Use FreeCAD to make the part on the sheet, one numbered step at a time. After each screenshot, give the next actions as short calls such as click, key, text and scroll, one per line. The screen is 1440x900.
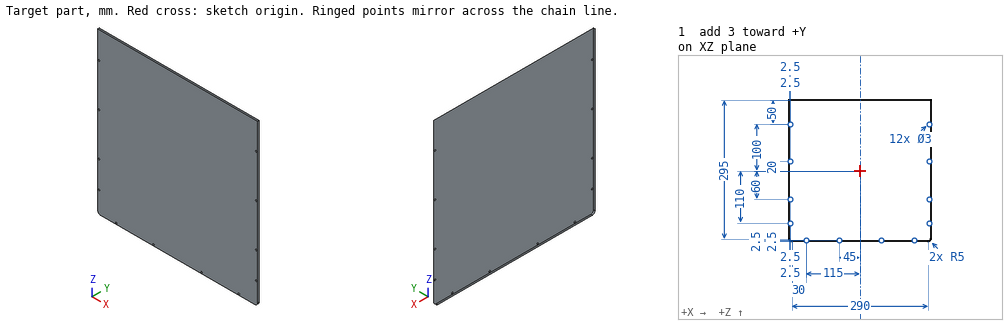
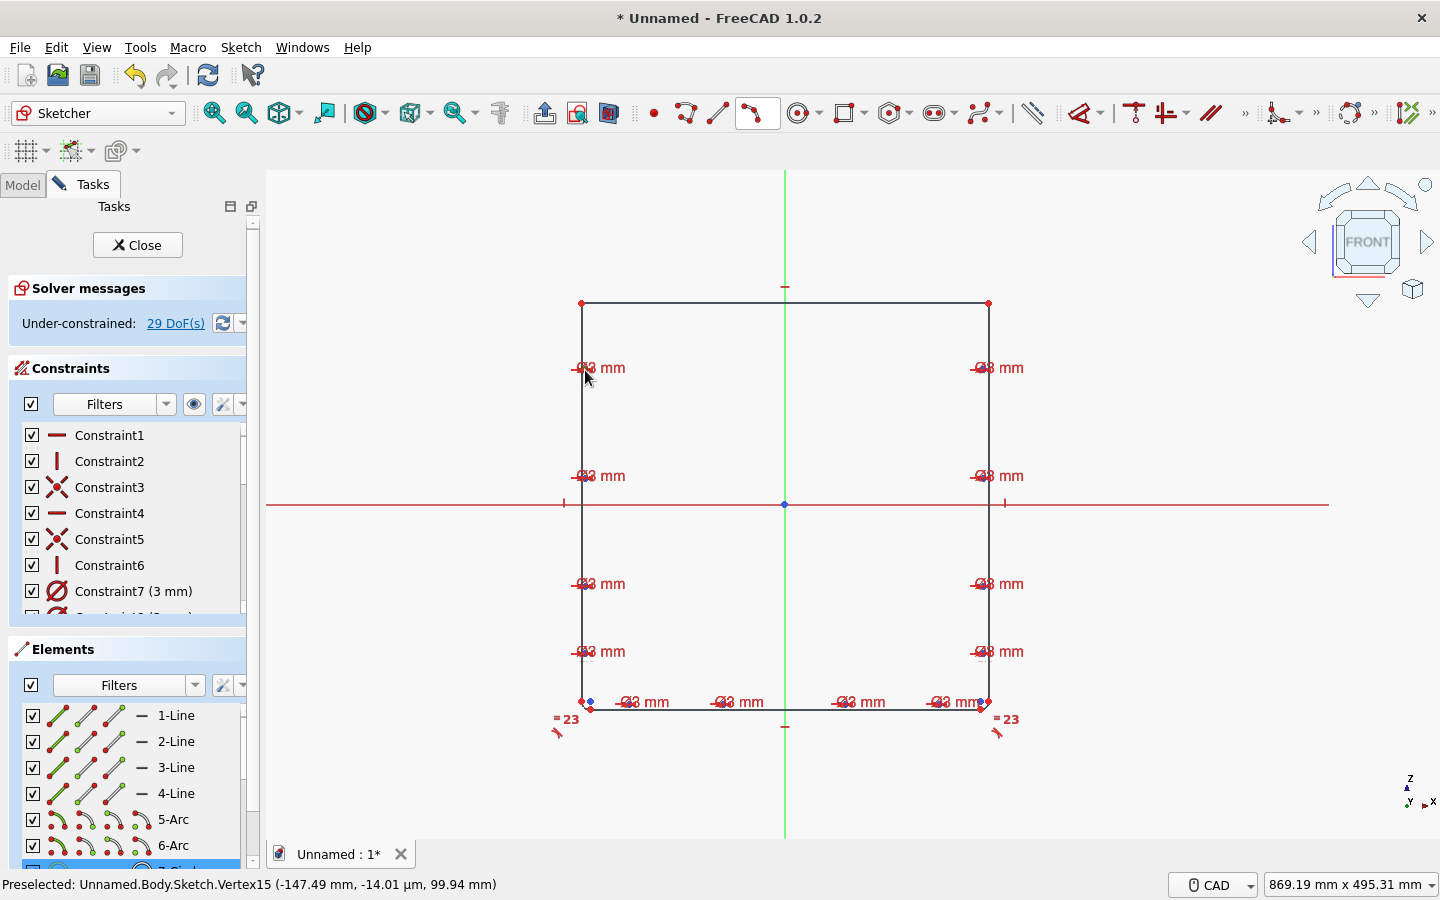
click(984, 370)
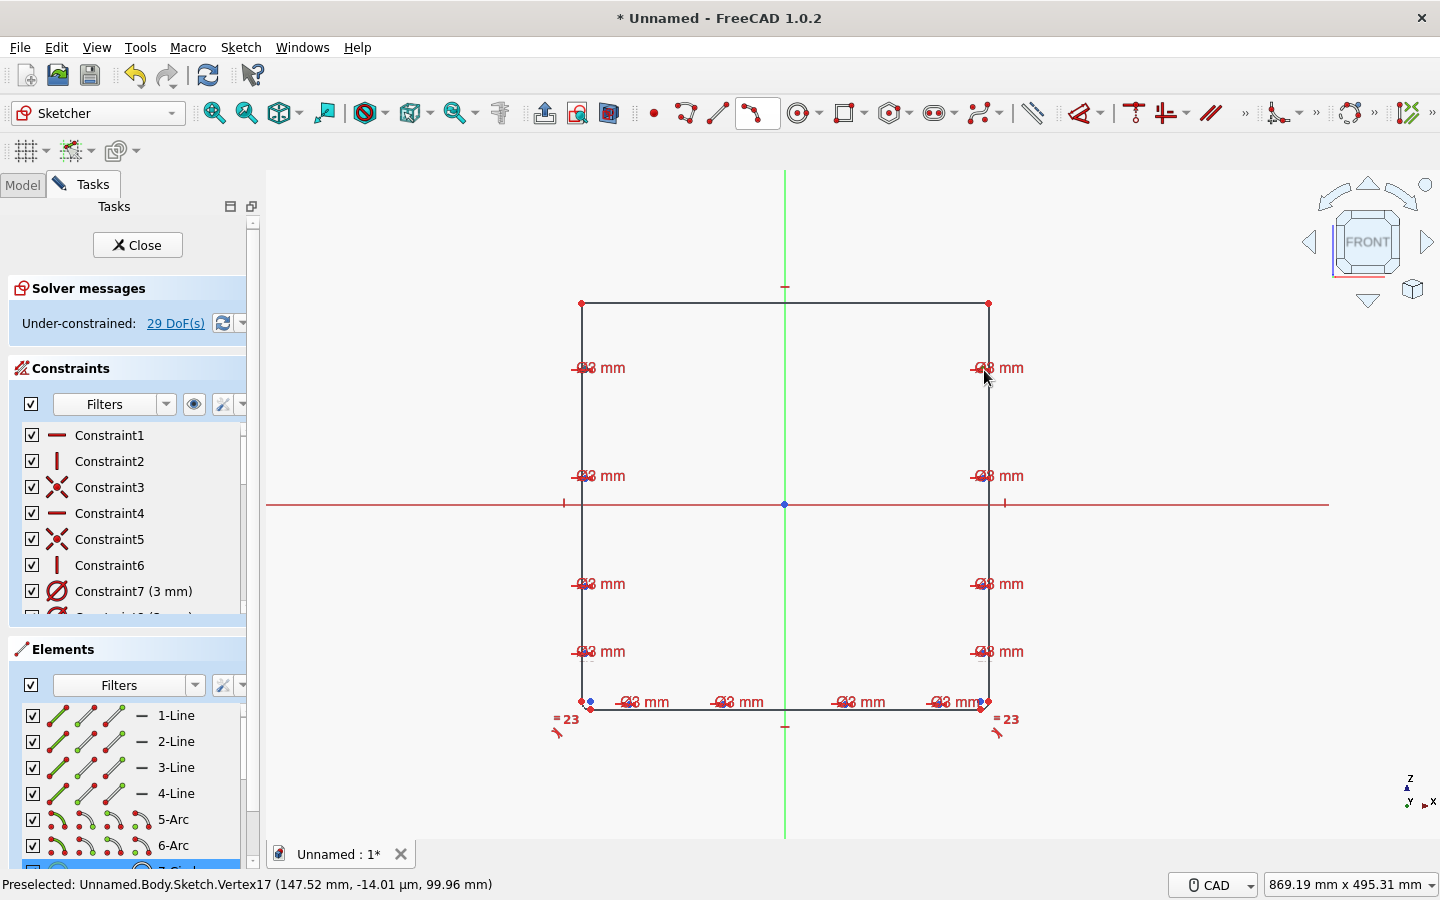
click(785, 767)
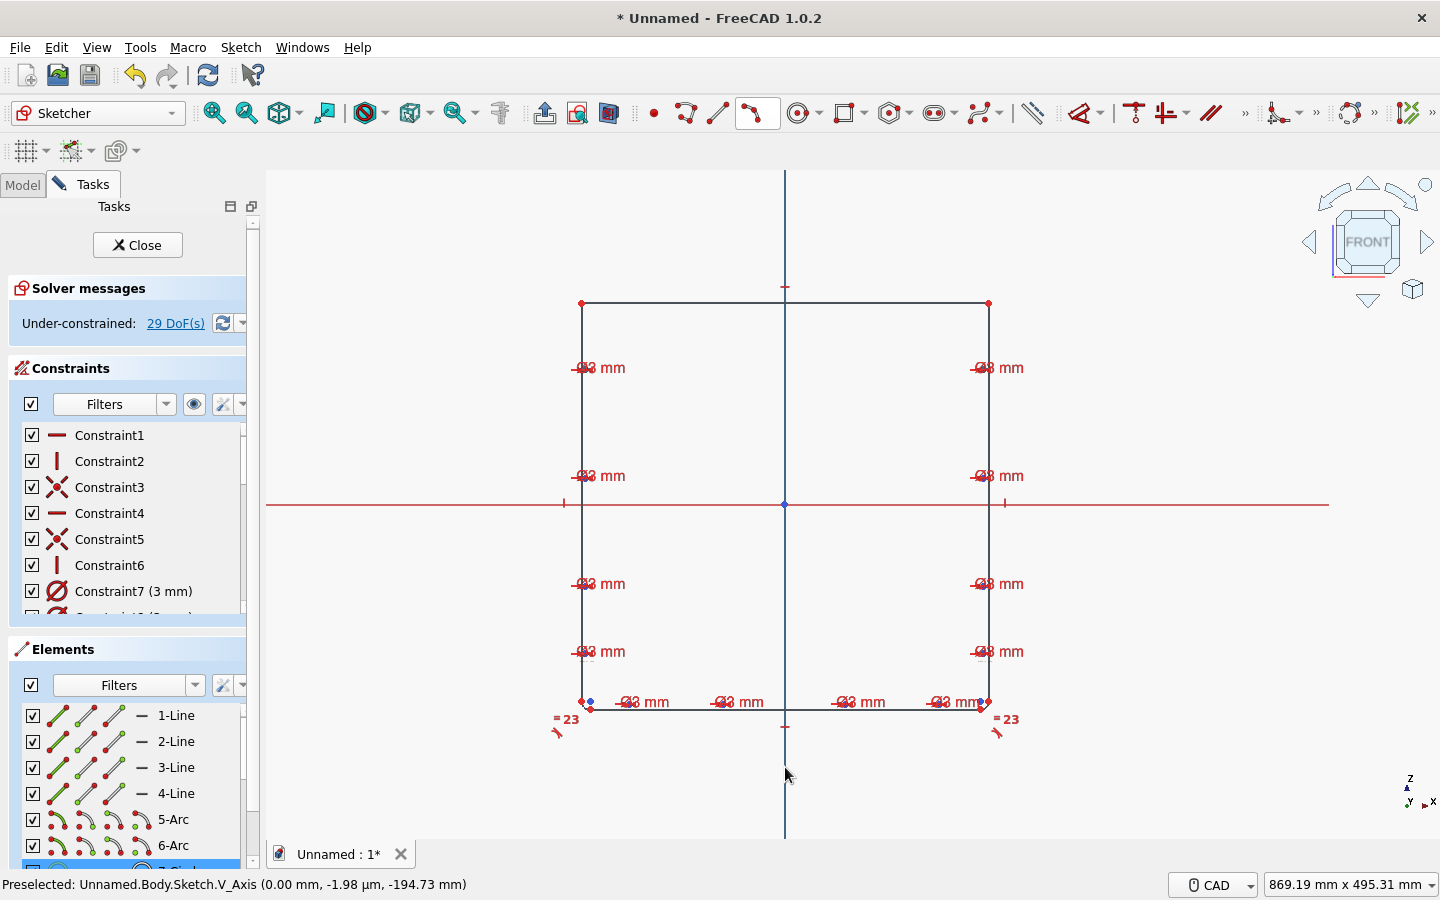
key(s)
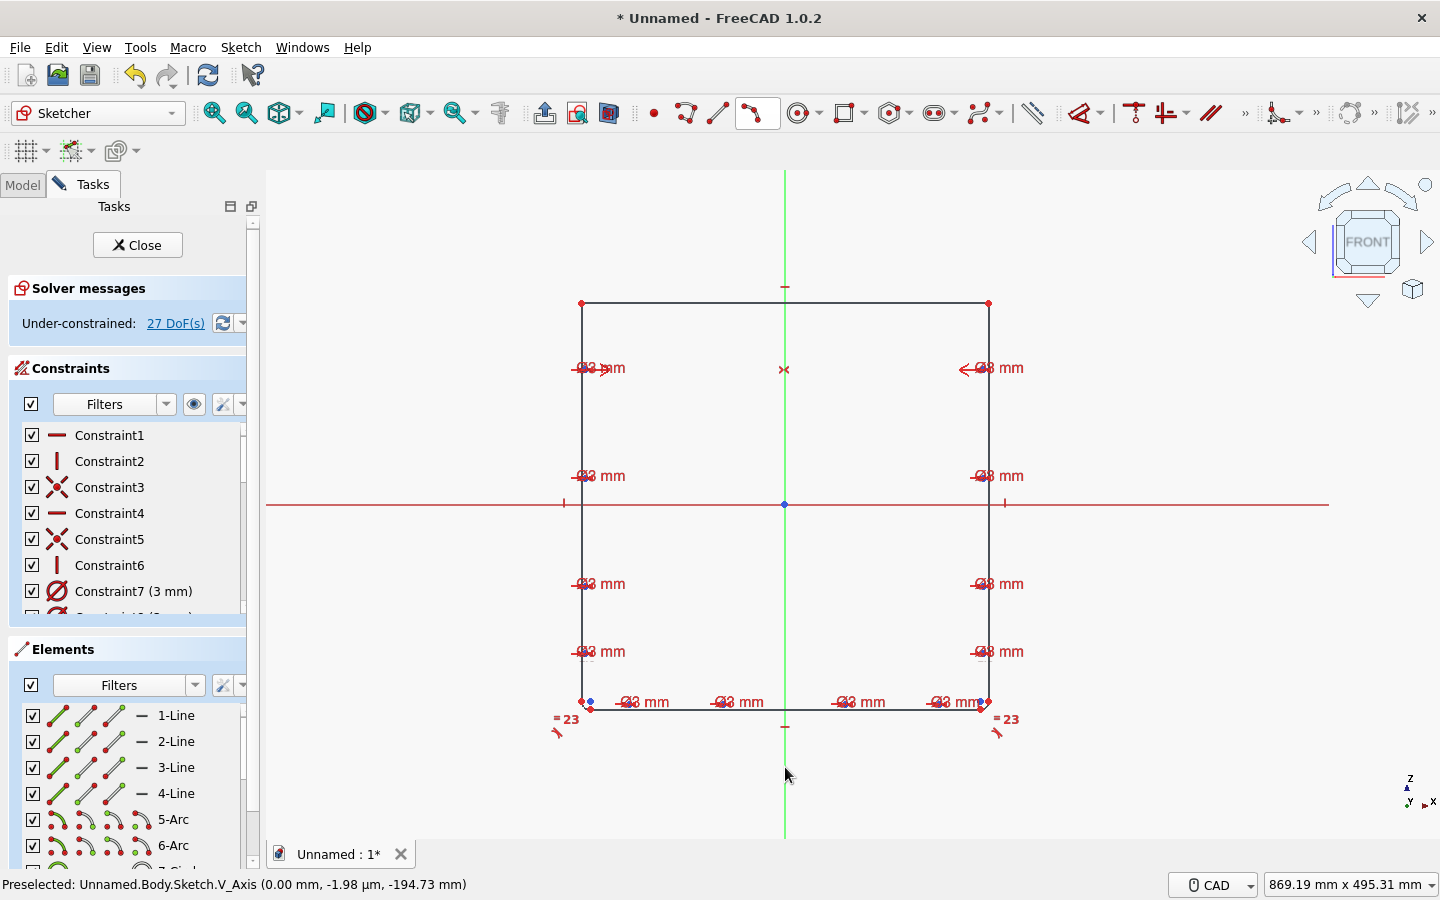
click(585, 478)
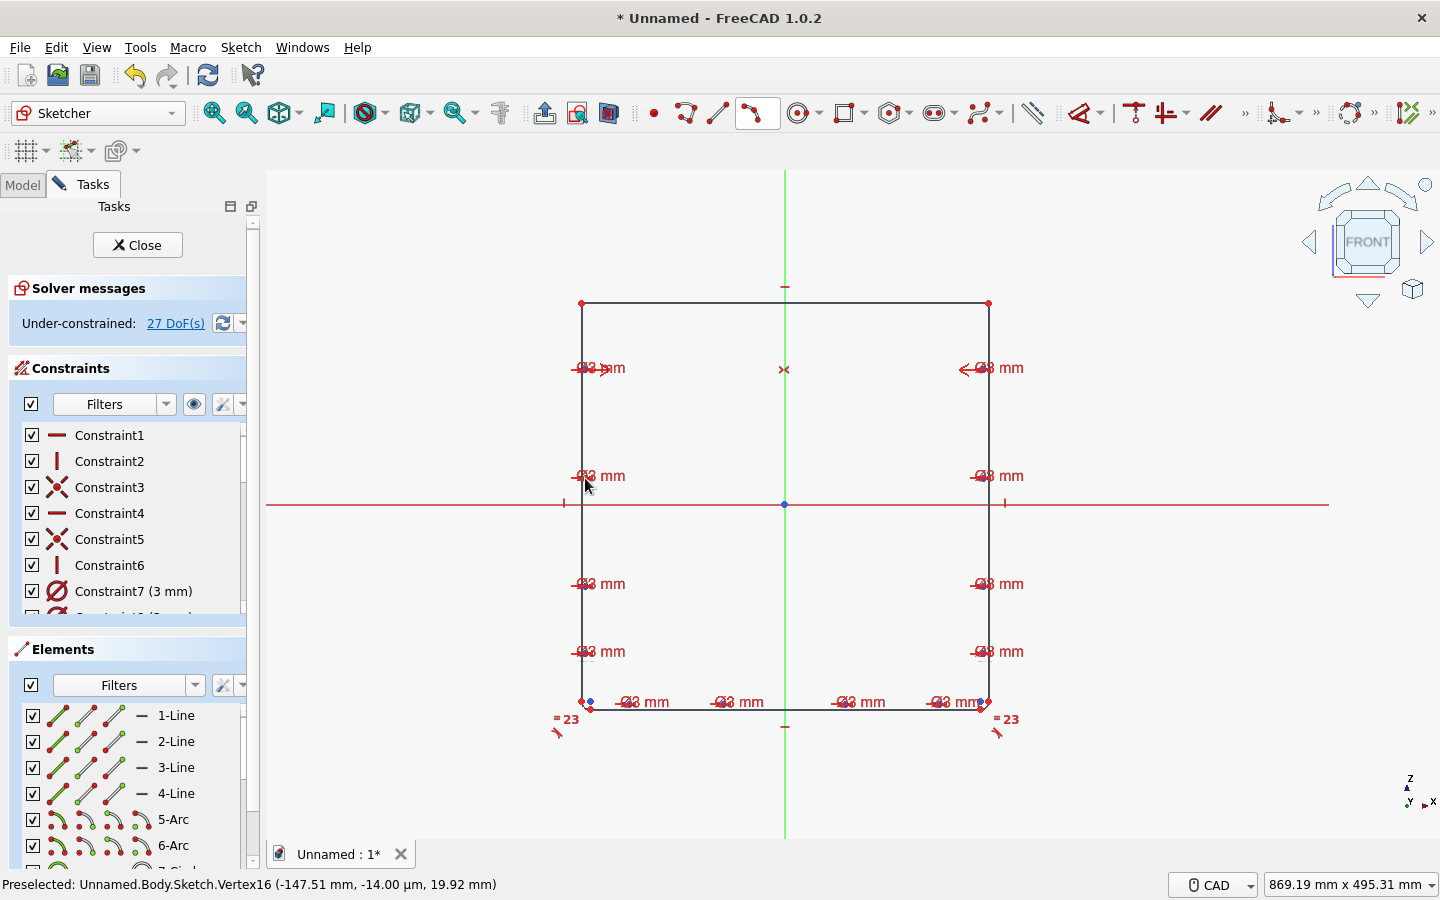
click(984, 478)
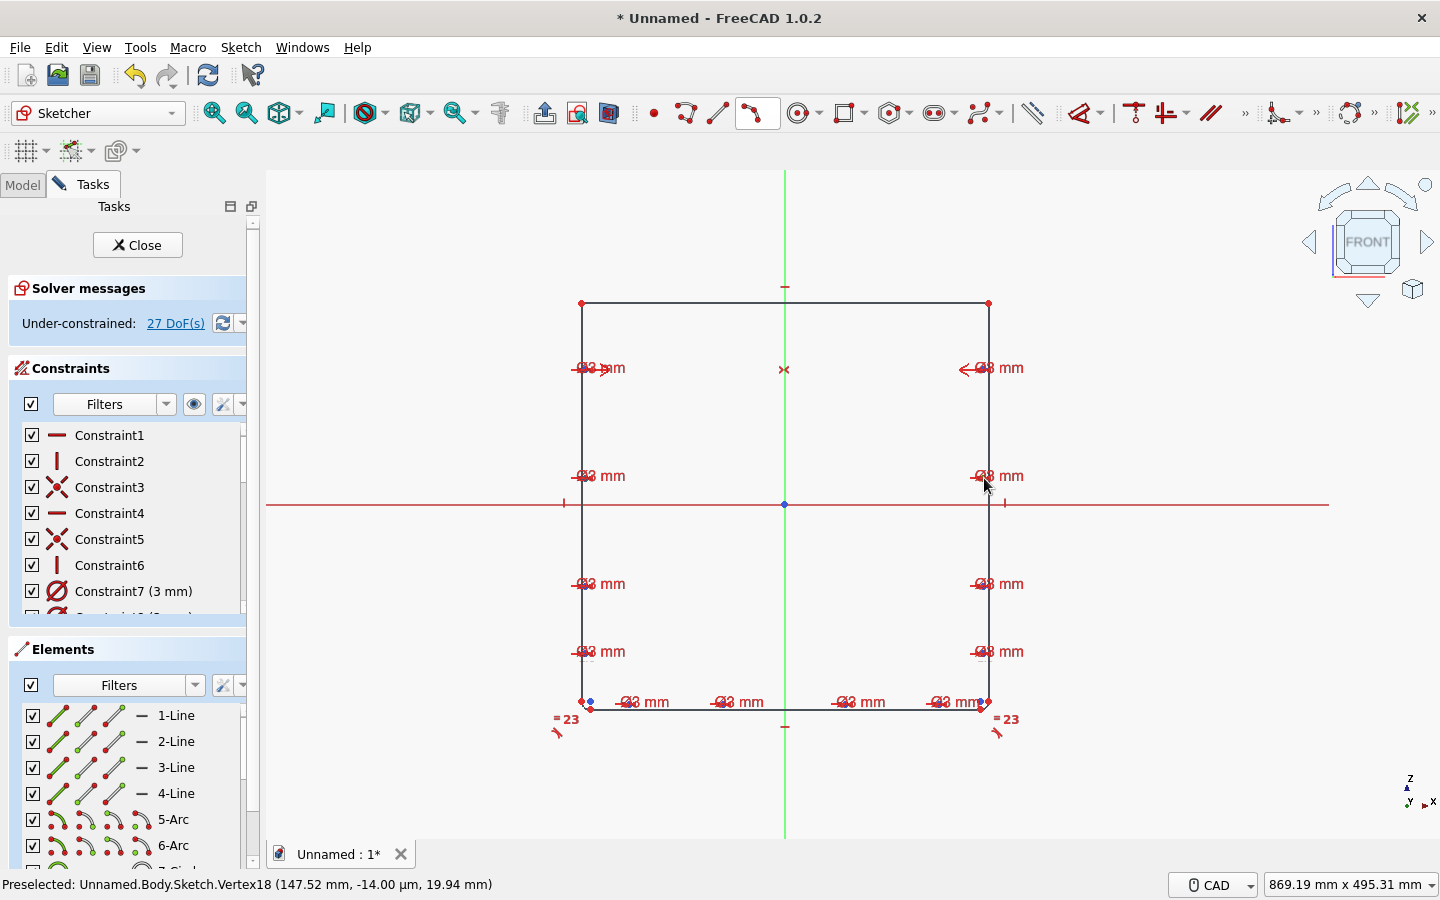
click(785, 767)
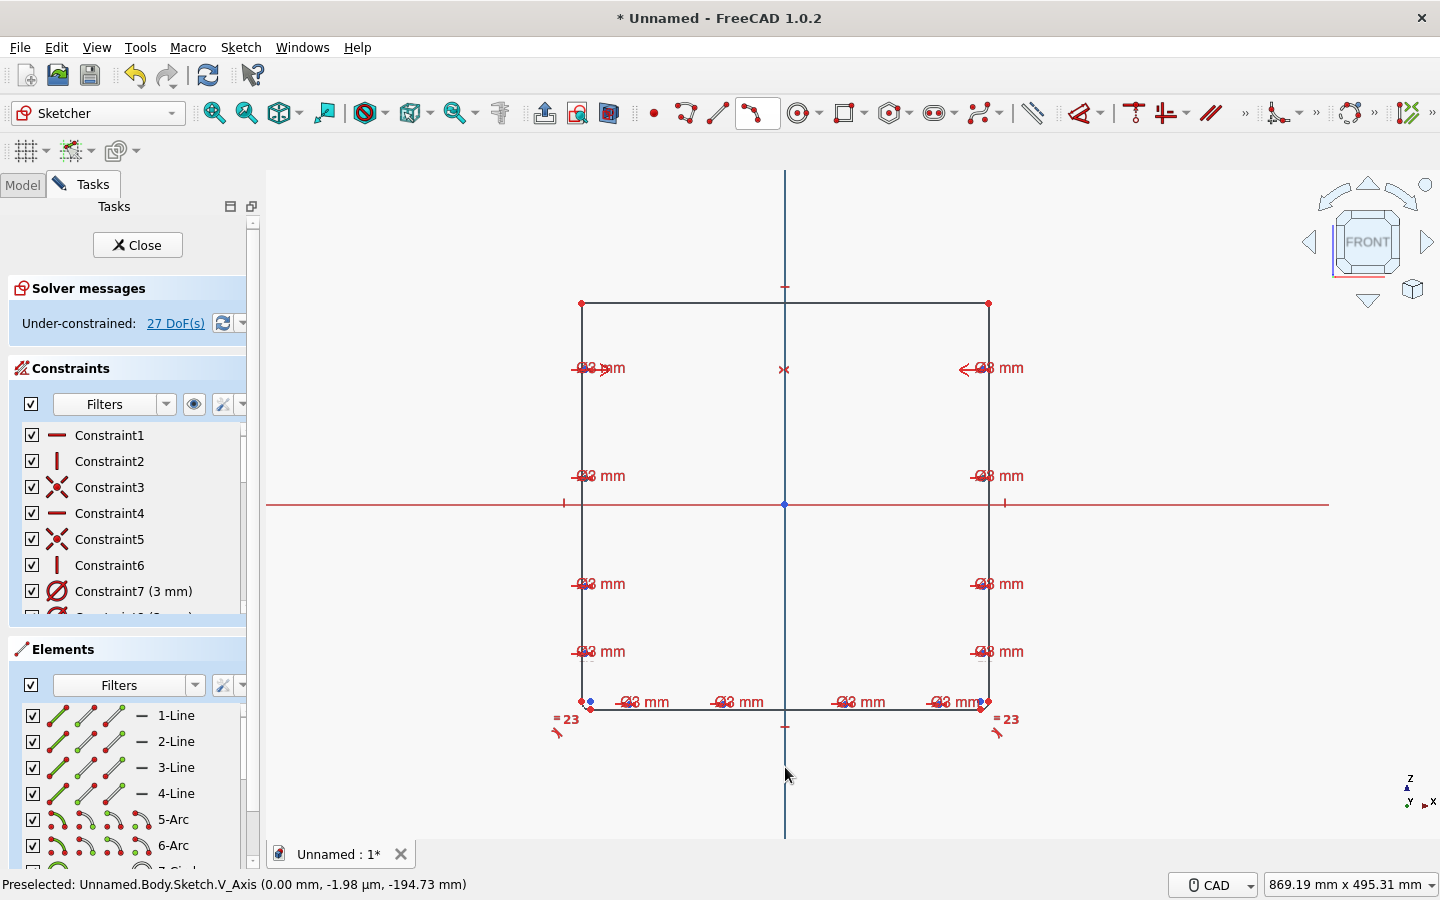
key(s)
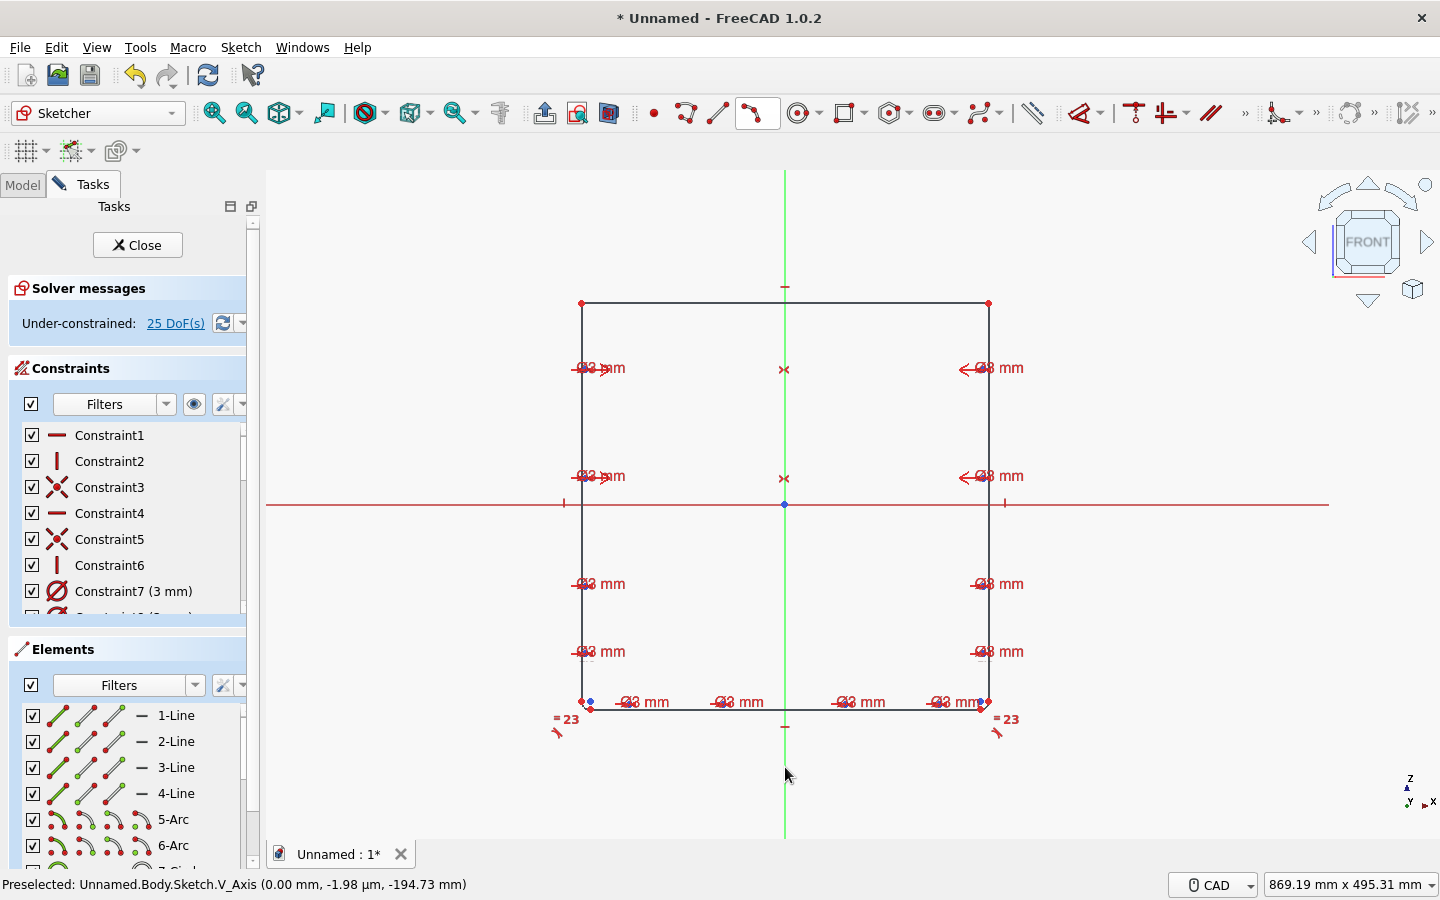
click(585, 586)